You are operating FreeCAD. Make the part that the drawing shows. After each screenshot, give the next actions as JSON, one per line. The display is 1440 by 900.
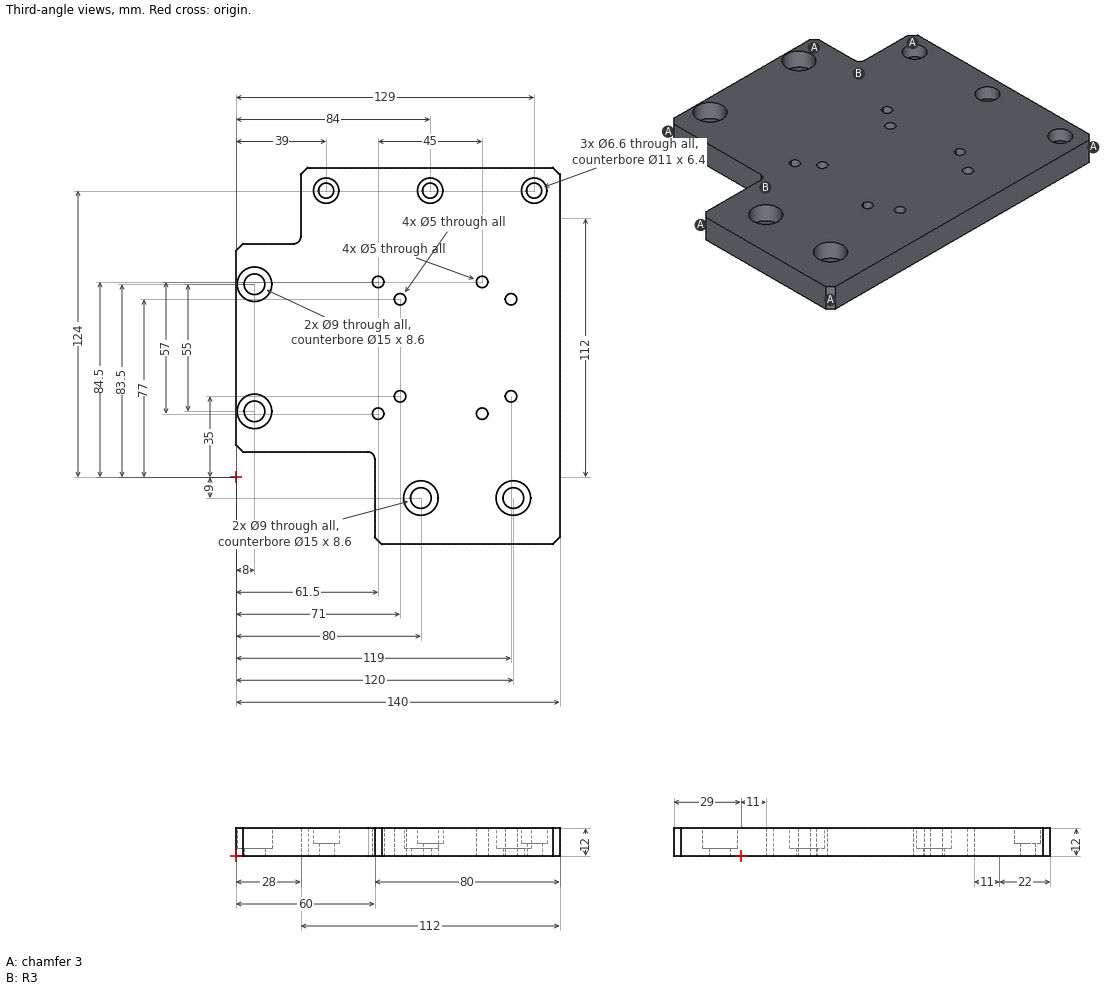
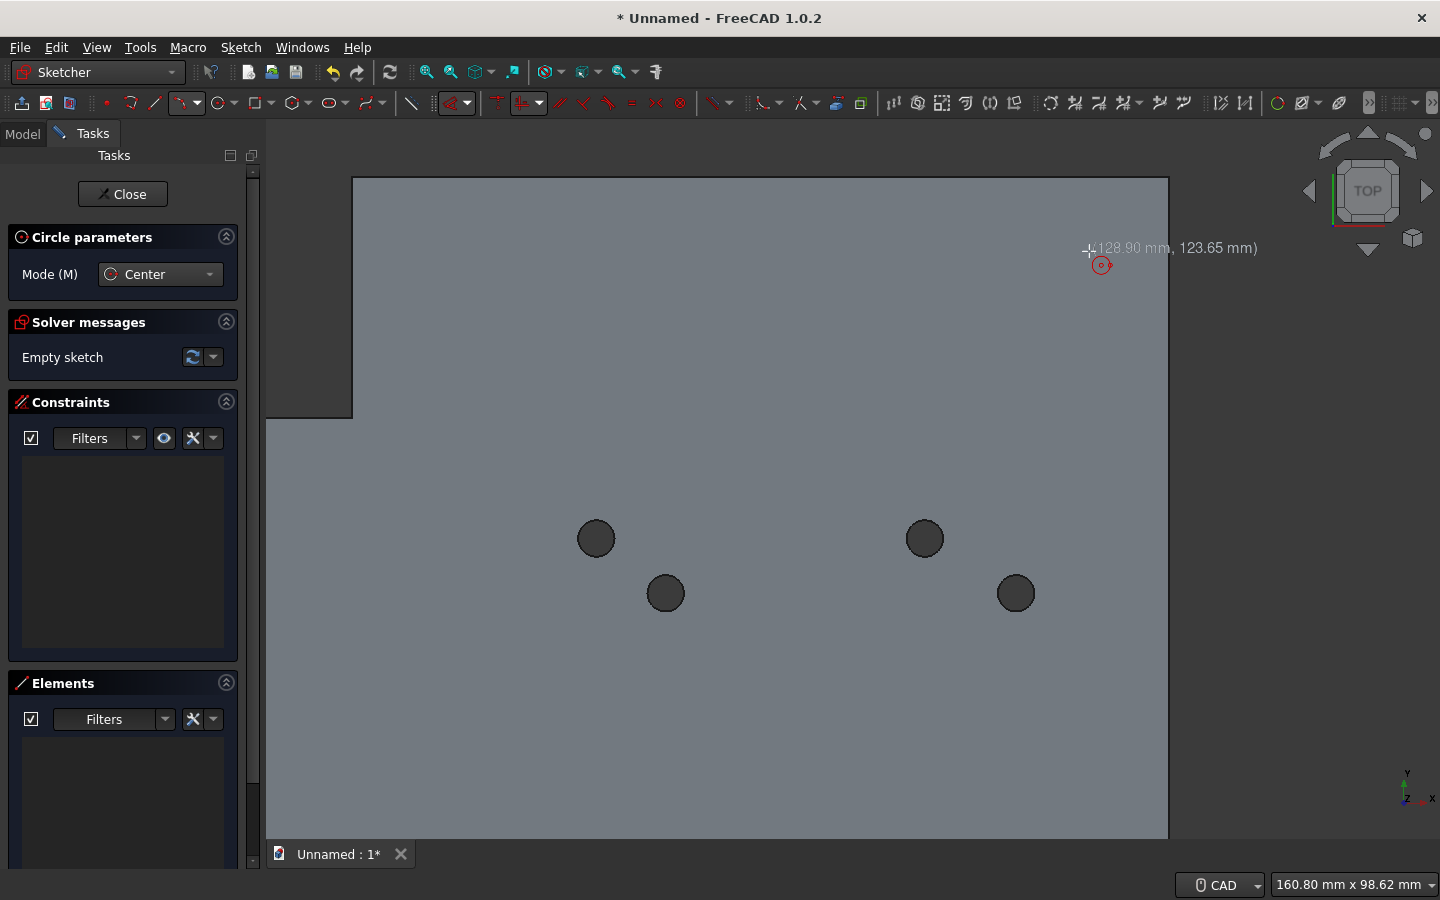
{"action": "left_click", "coordinate": [1089, 250]}
{"action": "mouse_move", "coordinate": [1106, 233]}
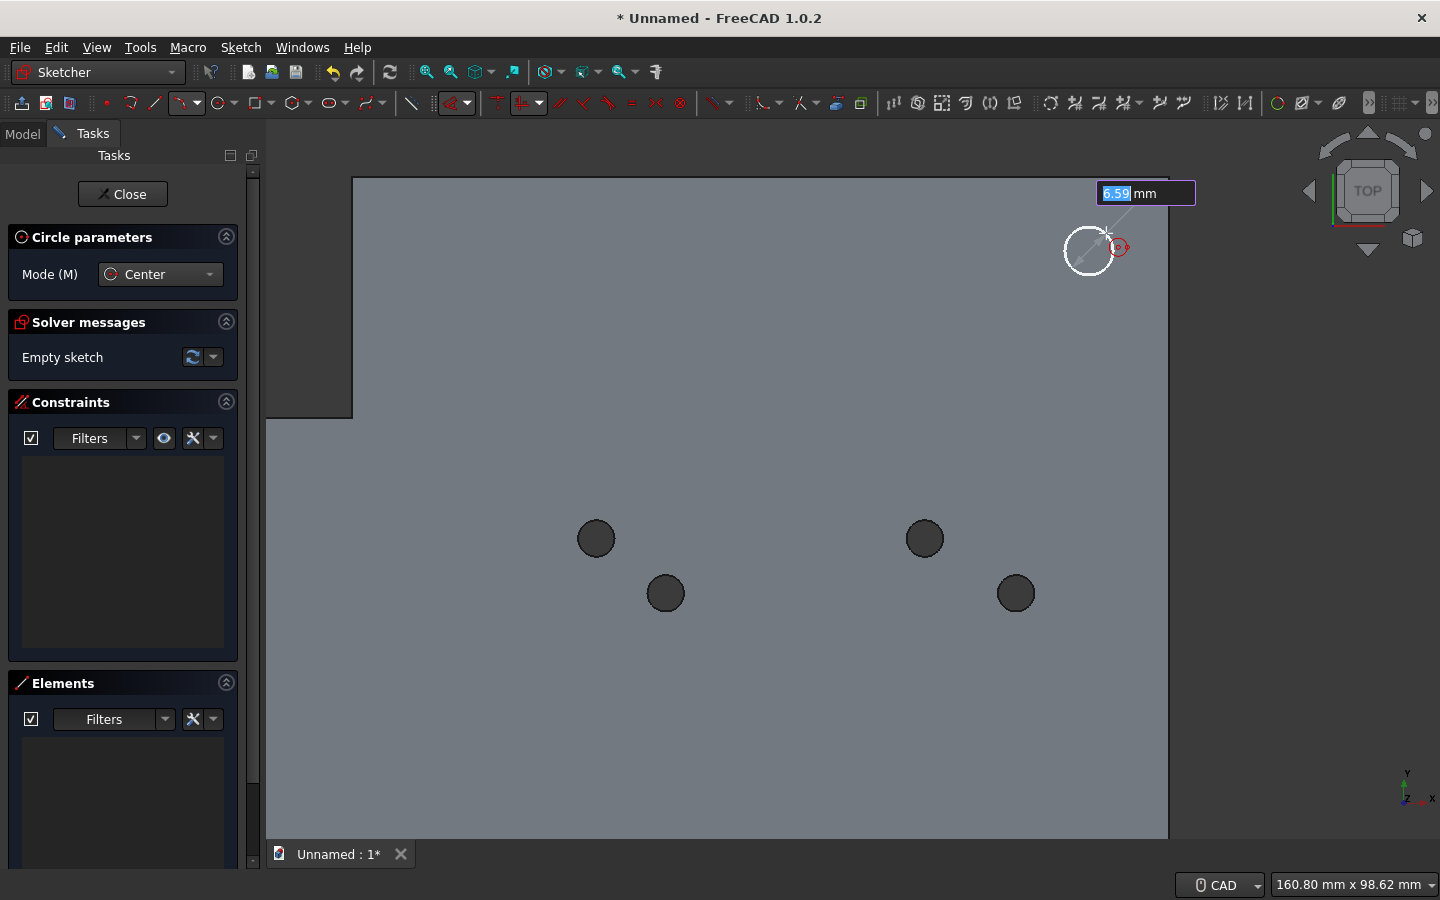
{"action": "type", "text": "6.6"}
{"action": "key", "text": "Return"}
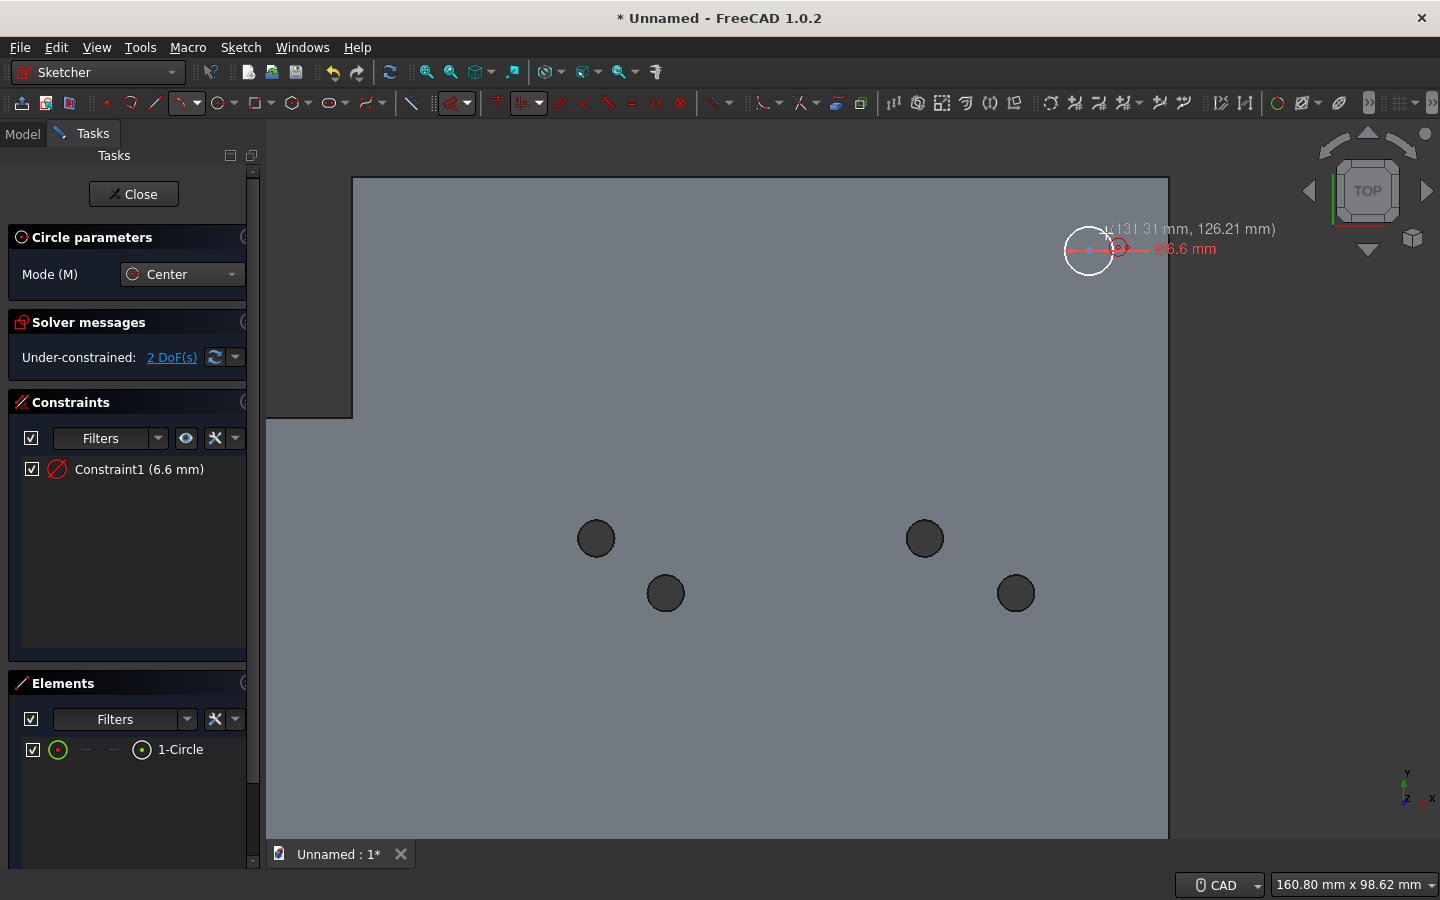
{"action": "left_click", "coordinate": [761, 250]}
{"action": "mouse_move", "coordinate": [778, 233]}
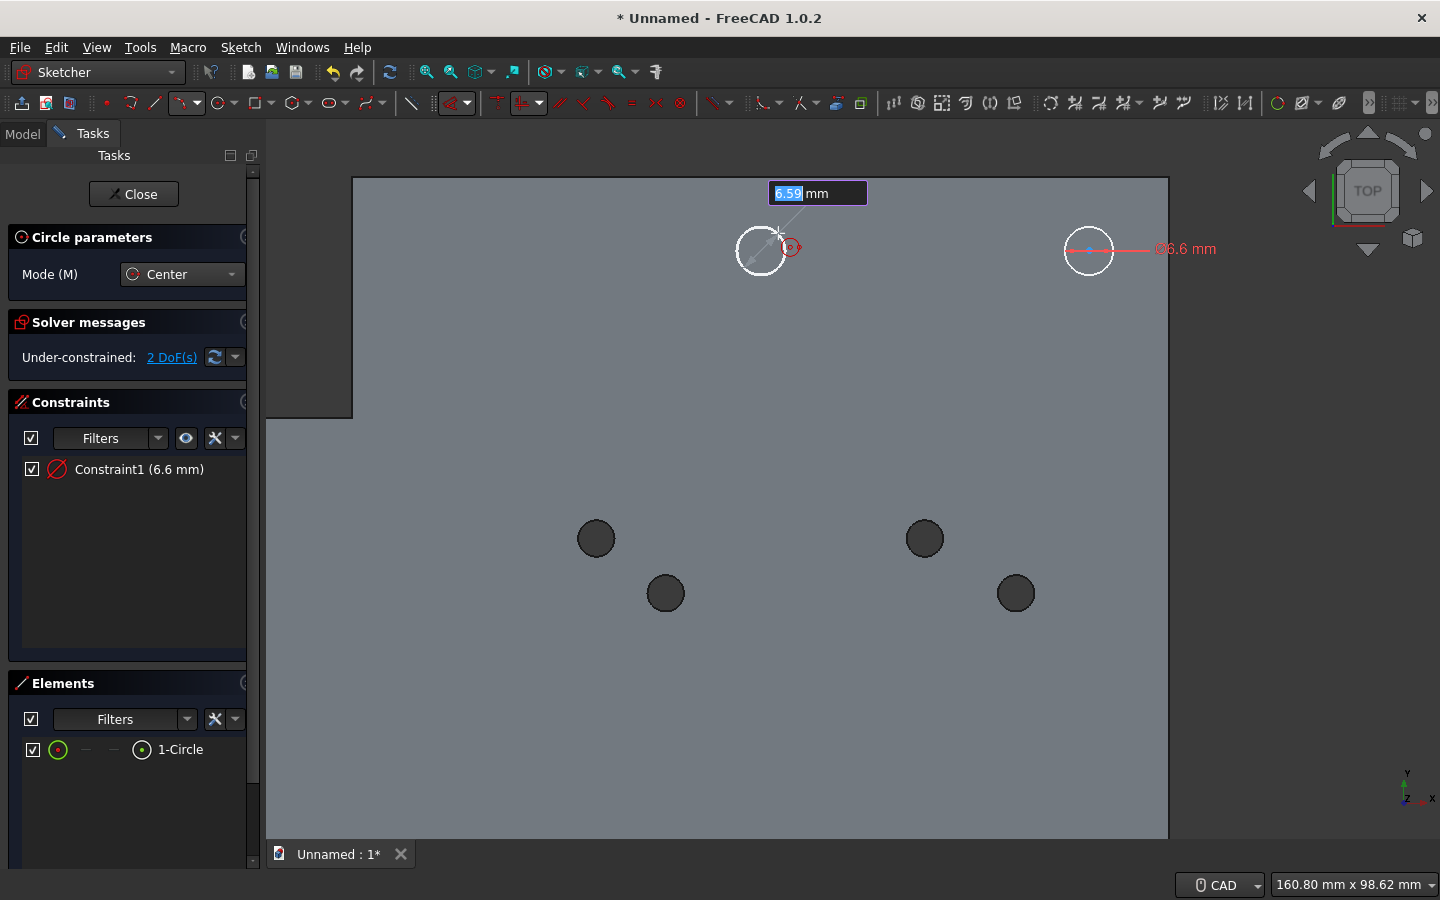
{"action": "type", "text": "6.6"}
{"action": "key", "text": "Return"}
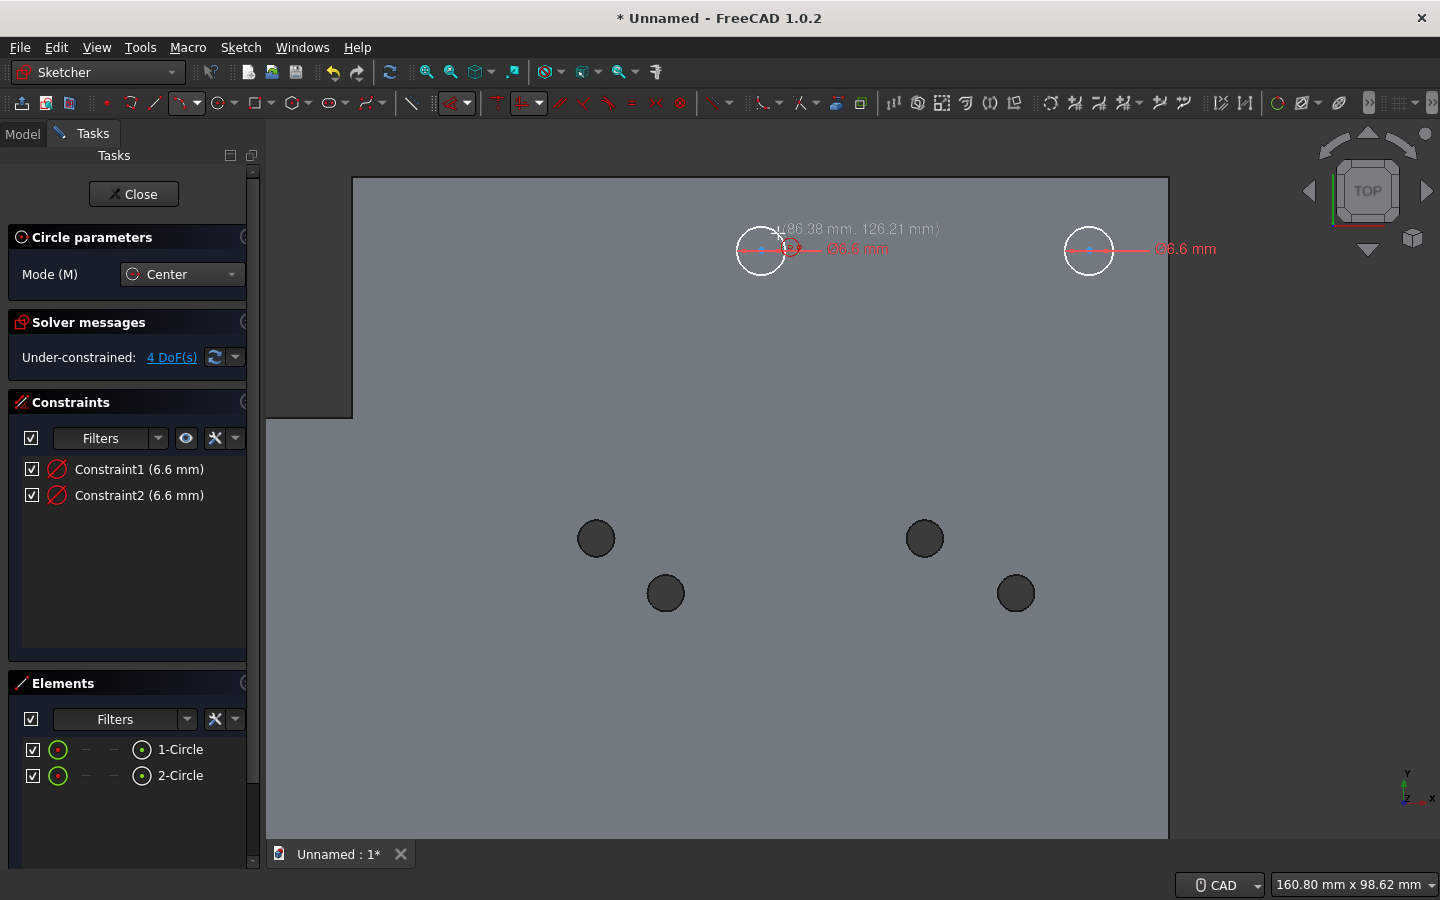
{"action": "left_click", "coordinate": [432, 250]}
{"action": "mouse_move", "coordinate": [449, 233]}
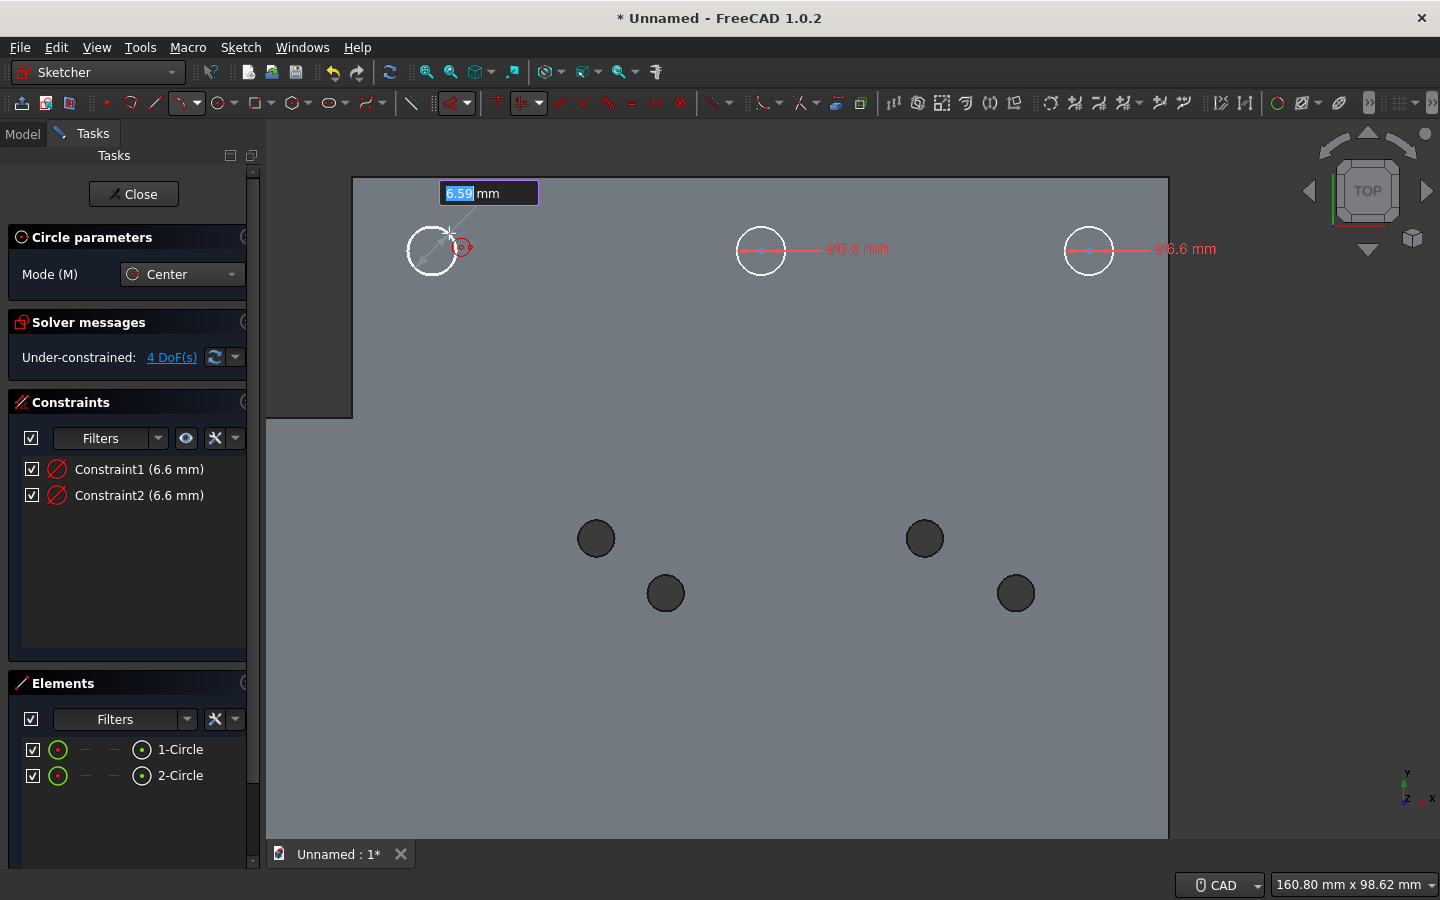
{"action": "type", "text": "6.6"}
{"action": "key", "text": "Return"}
{"action": "key", "text": "Escape"}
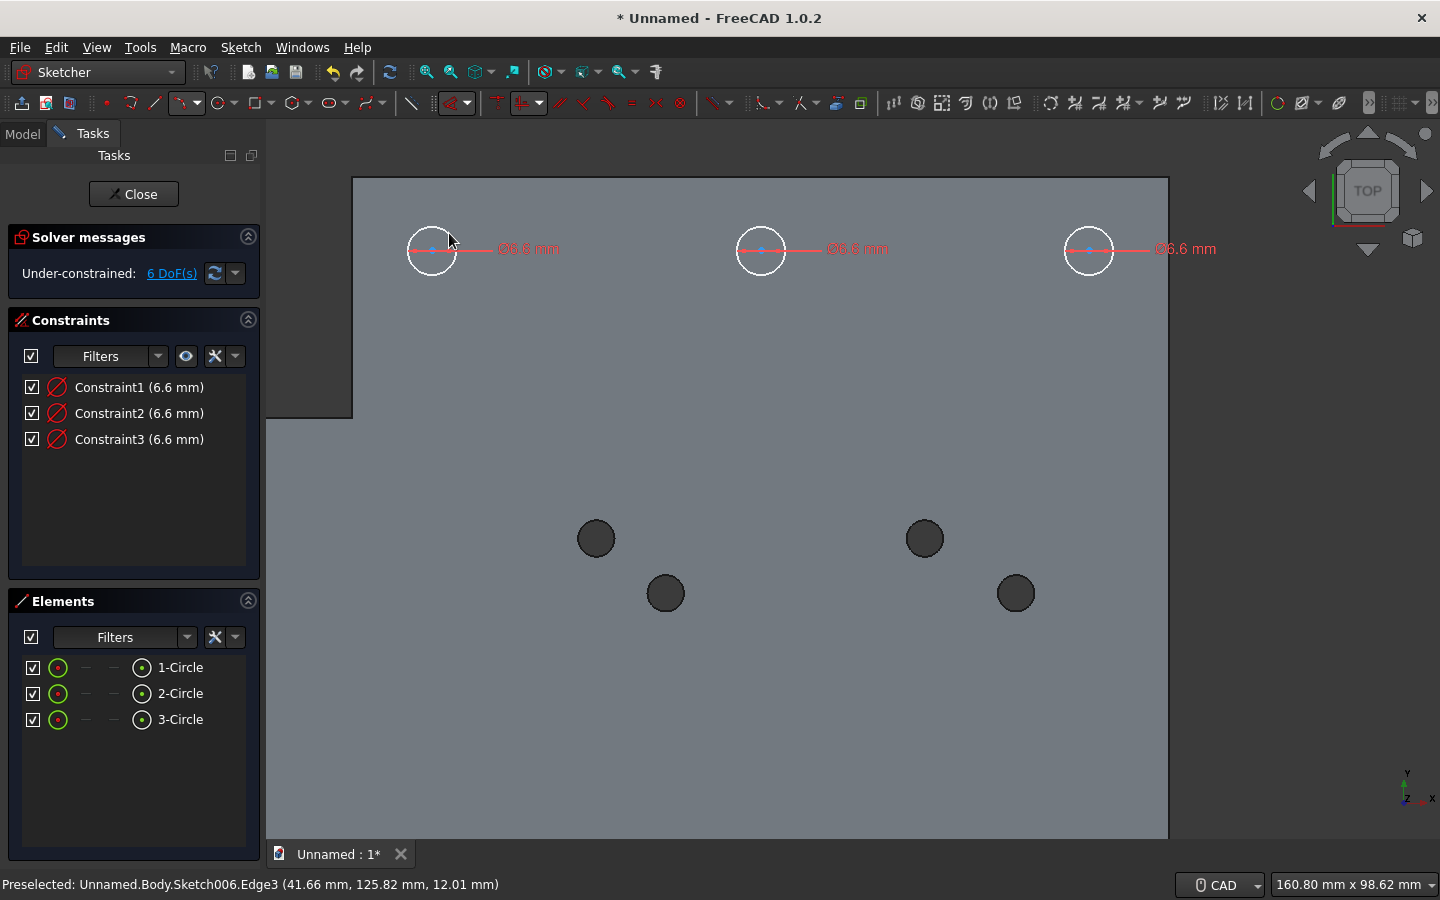
{"action": "left_click", "coordinate": [761, 251]}